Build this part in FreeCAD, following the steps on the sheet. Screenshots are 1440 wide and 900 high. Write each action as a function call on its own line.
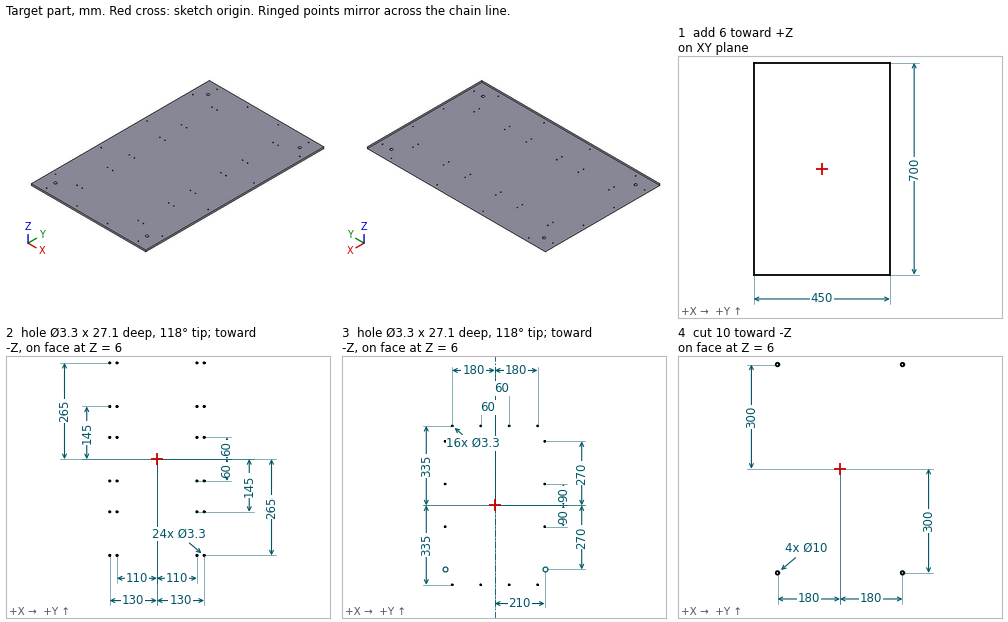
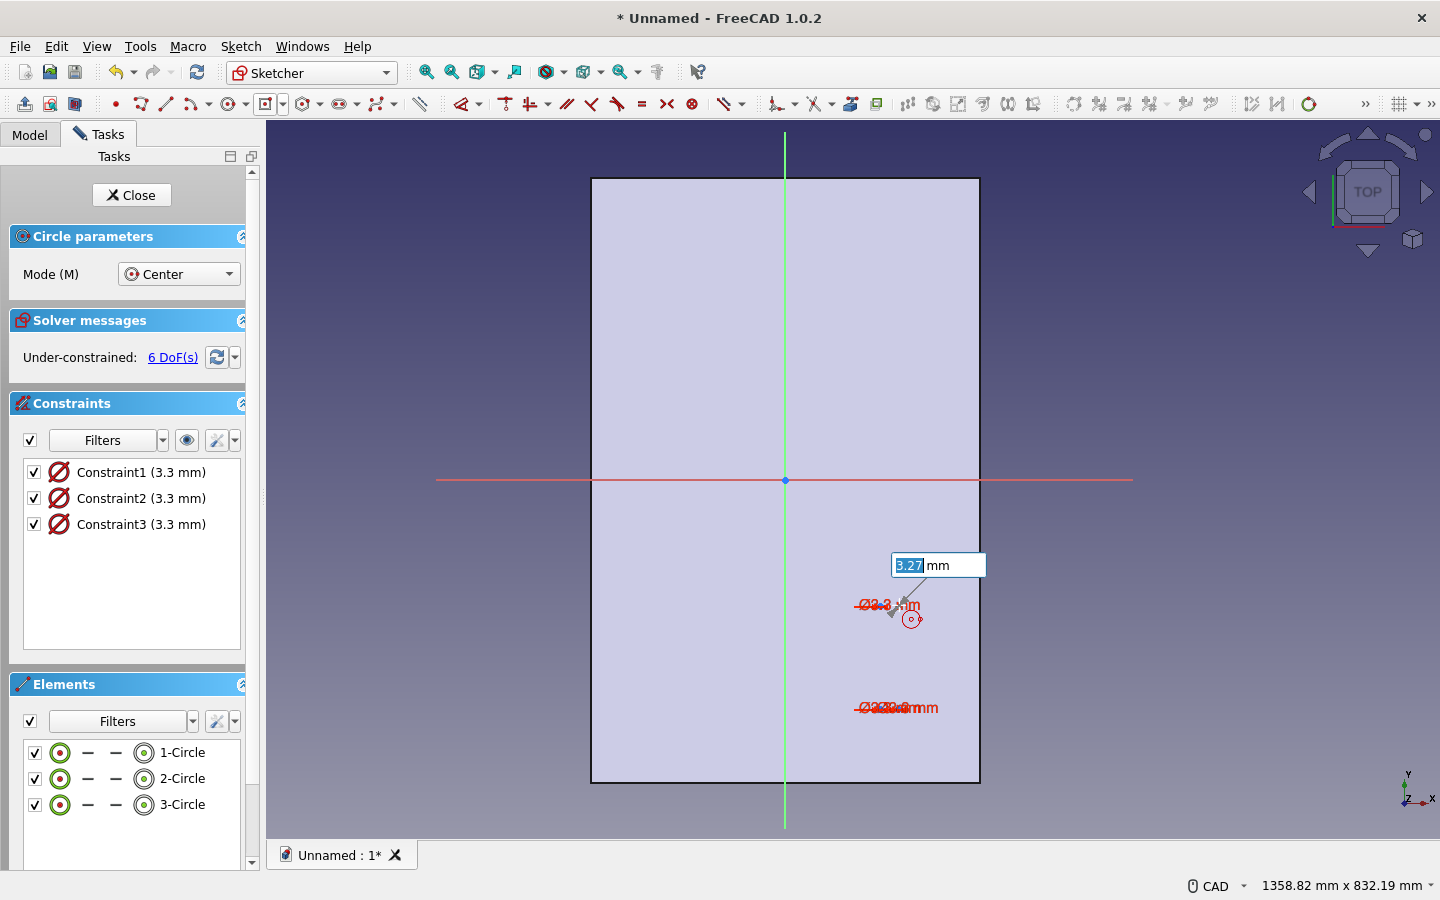
text(3.3)
key(Return)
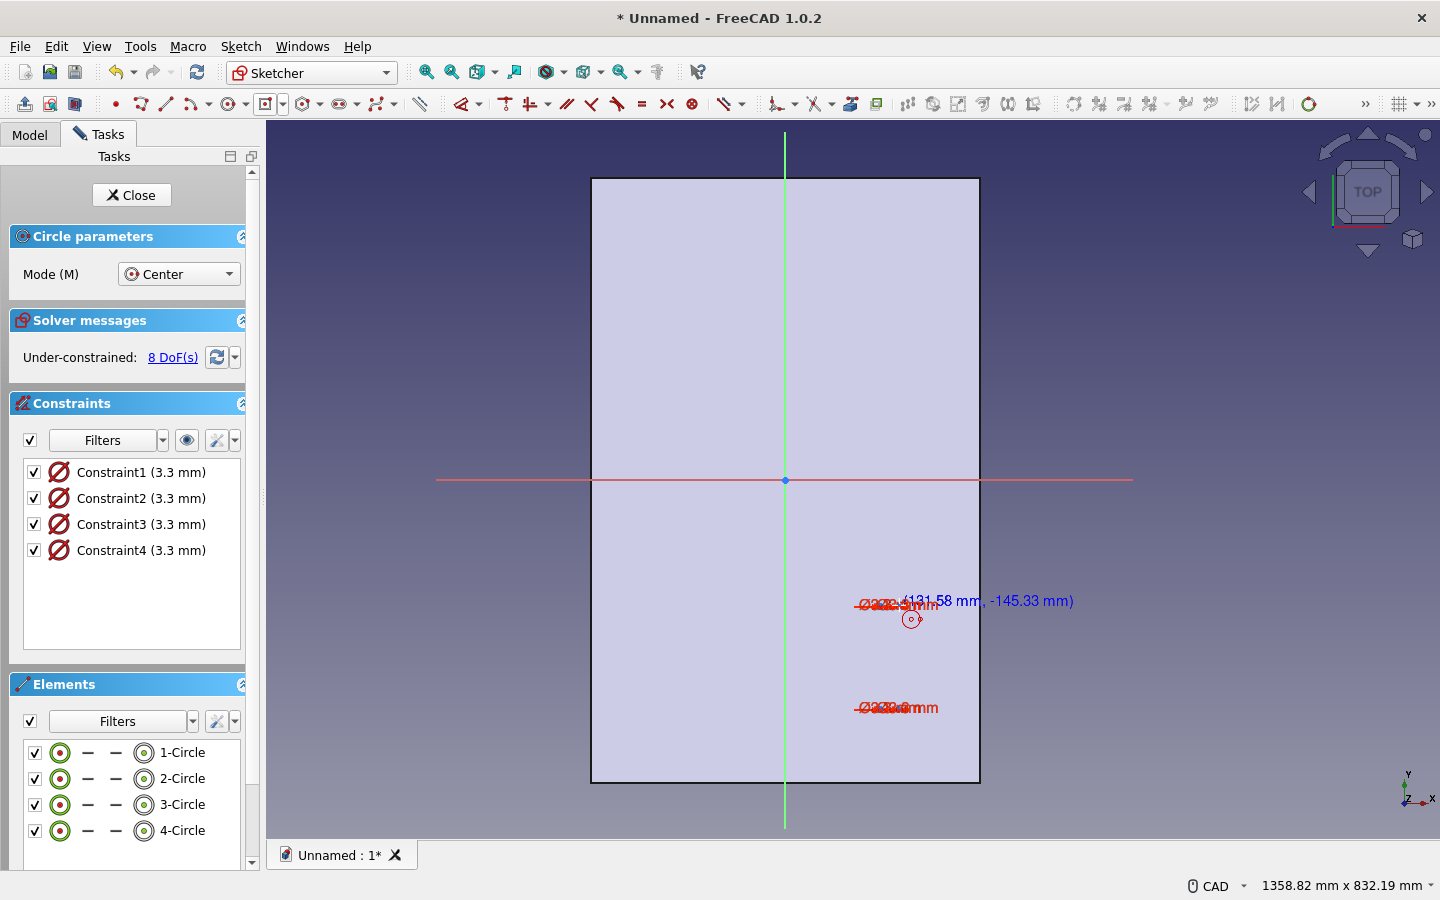
scroll(880, 532, up, 14)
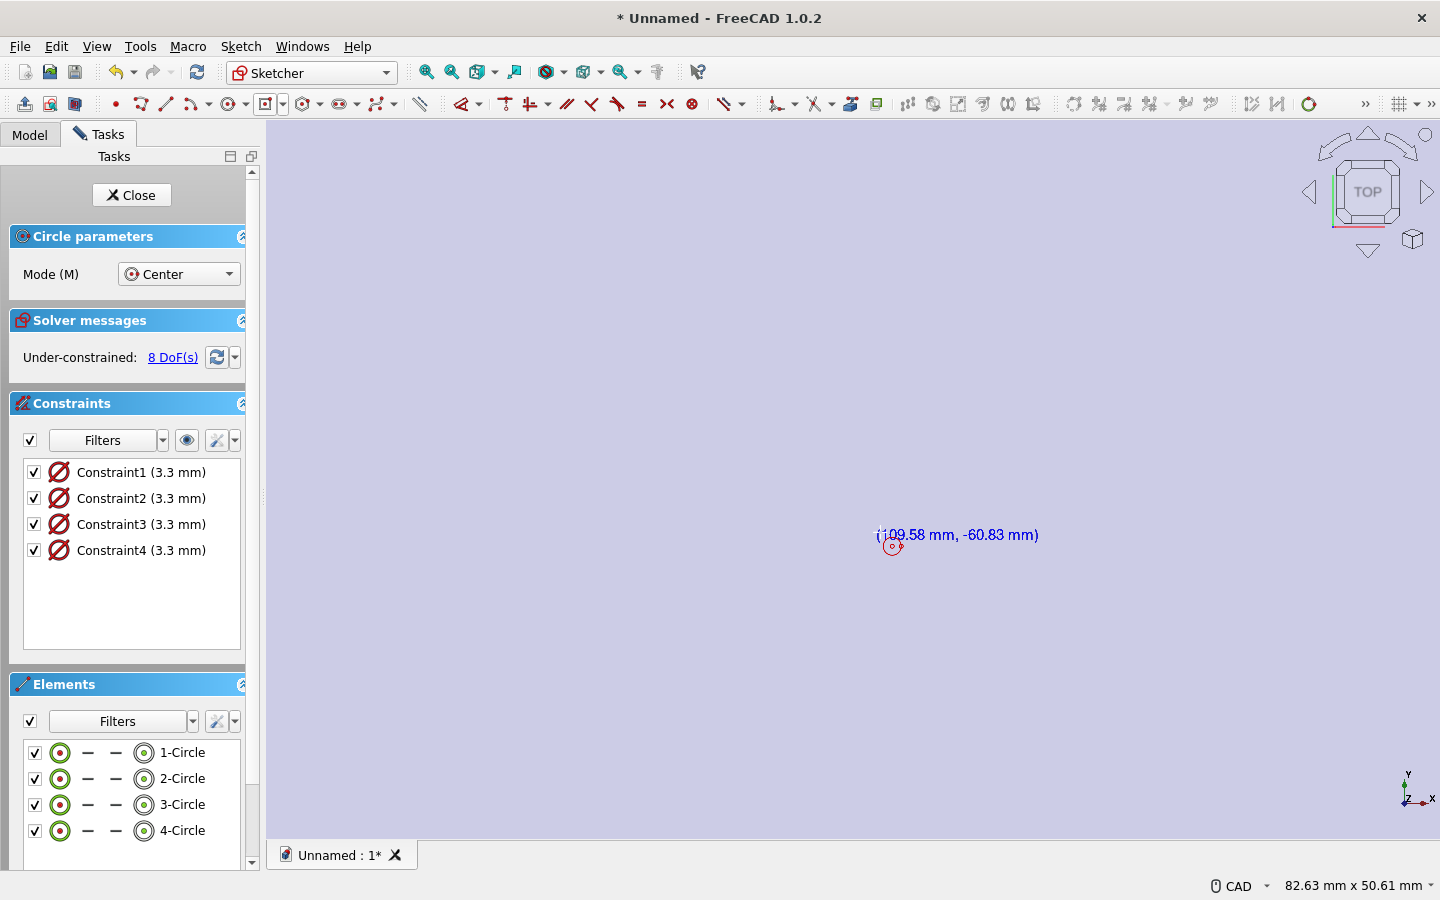
scroll(880, 532, down, 14)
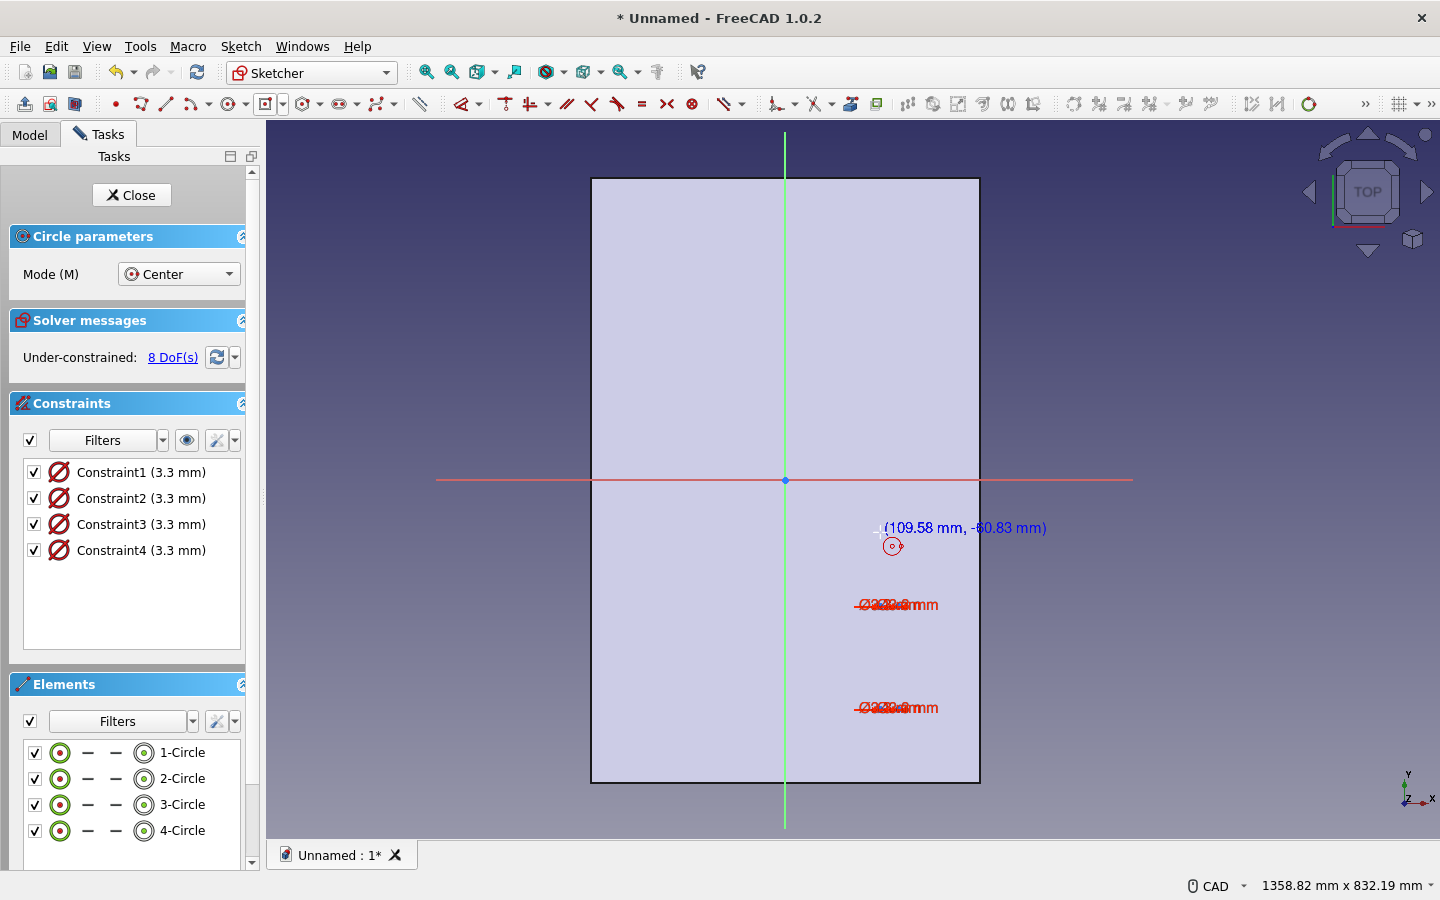
click(880, 532)
move(881, 531)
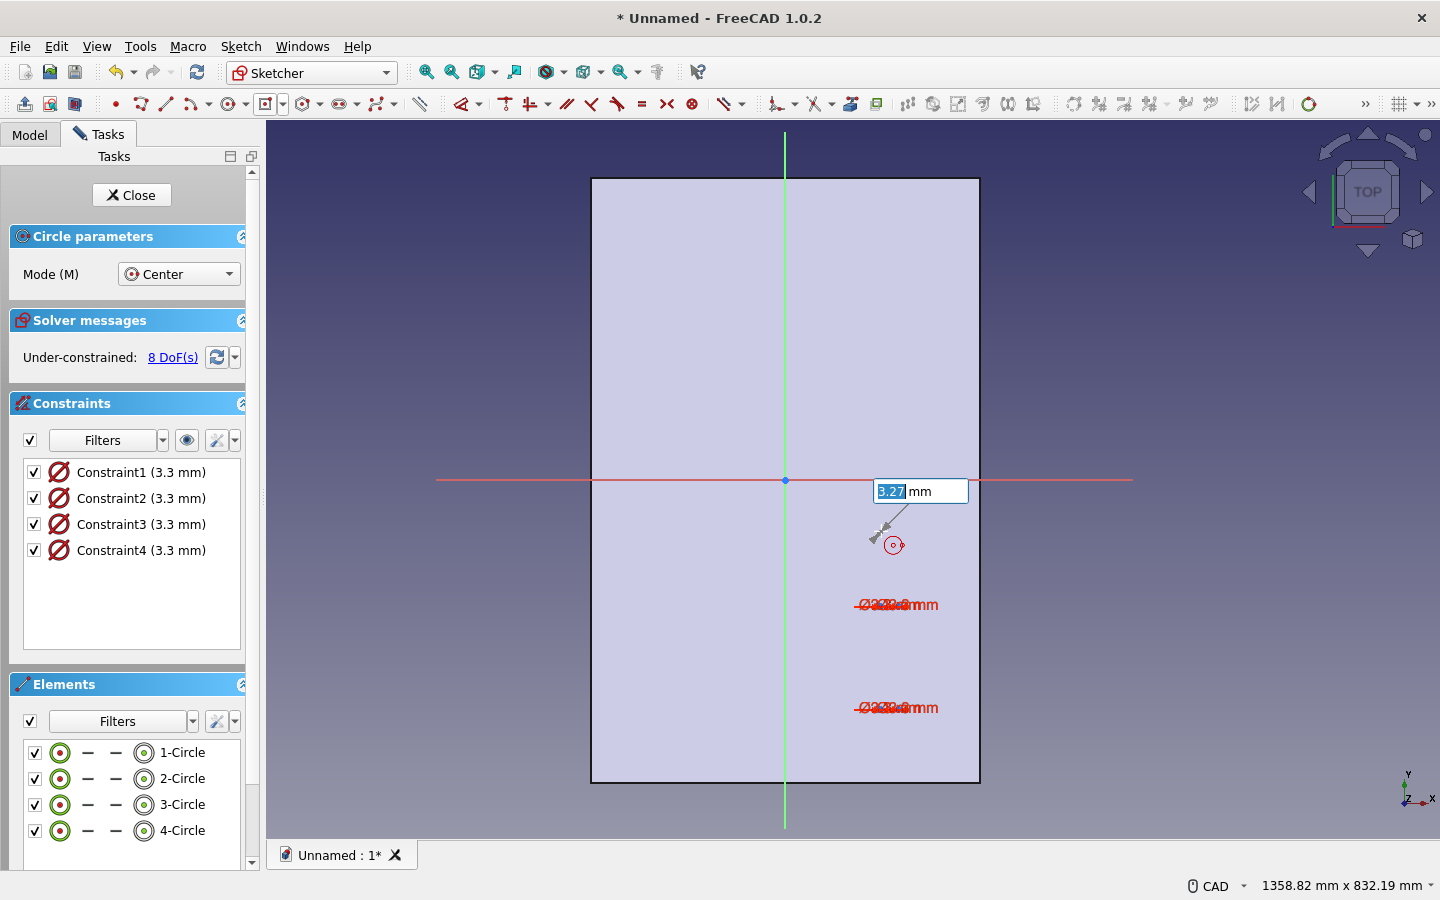
text(3.3)
key(Return)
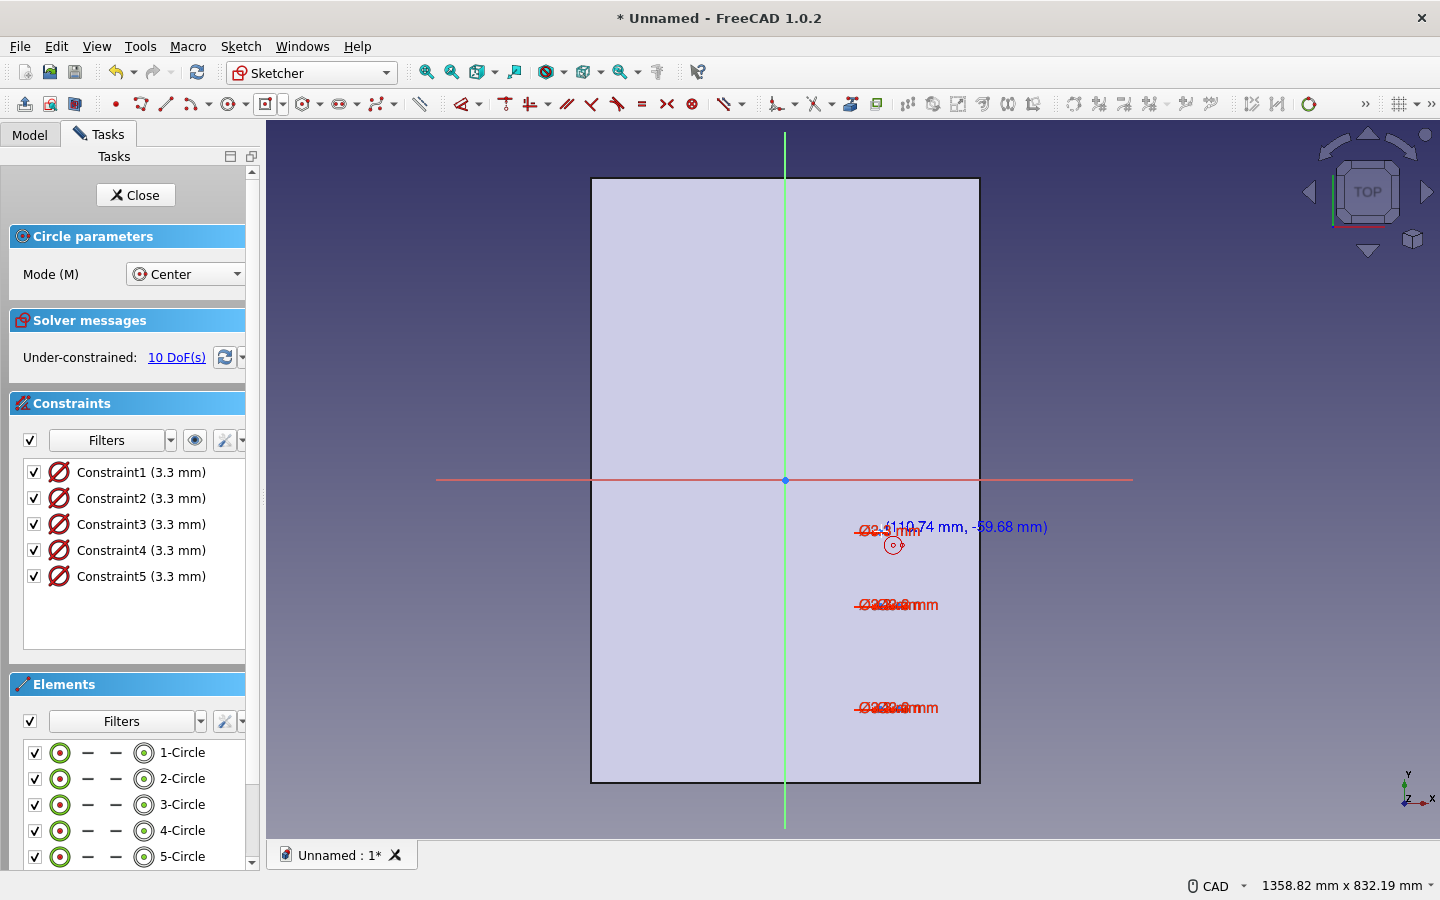
scroll(898, 532, up, 14)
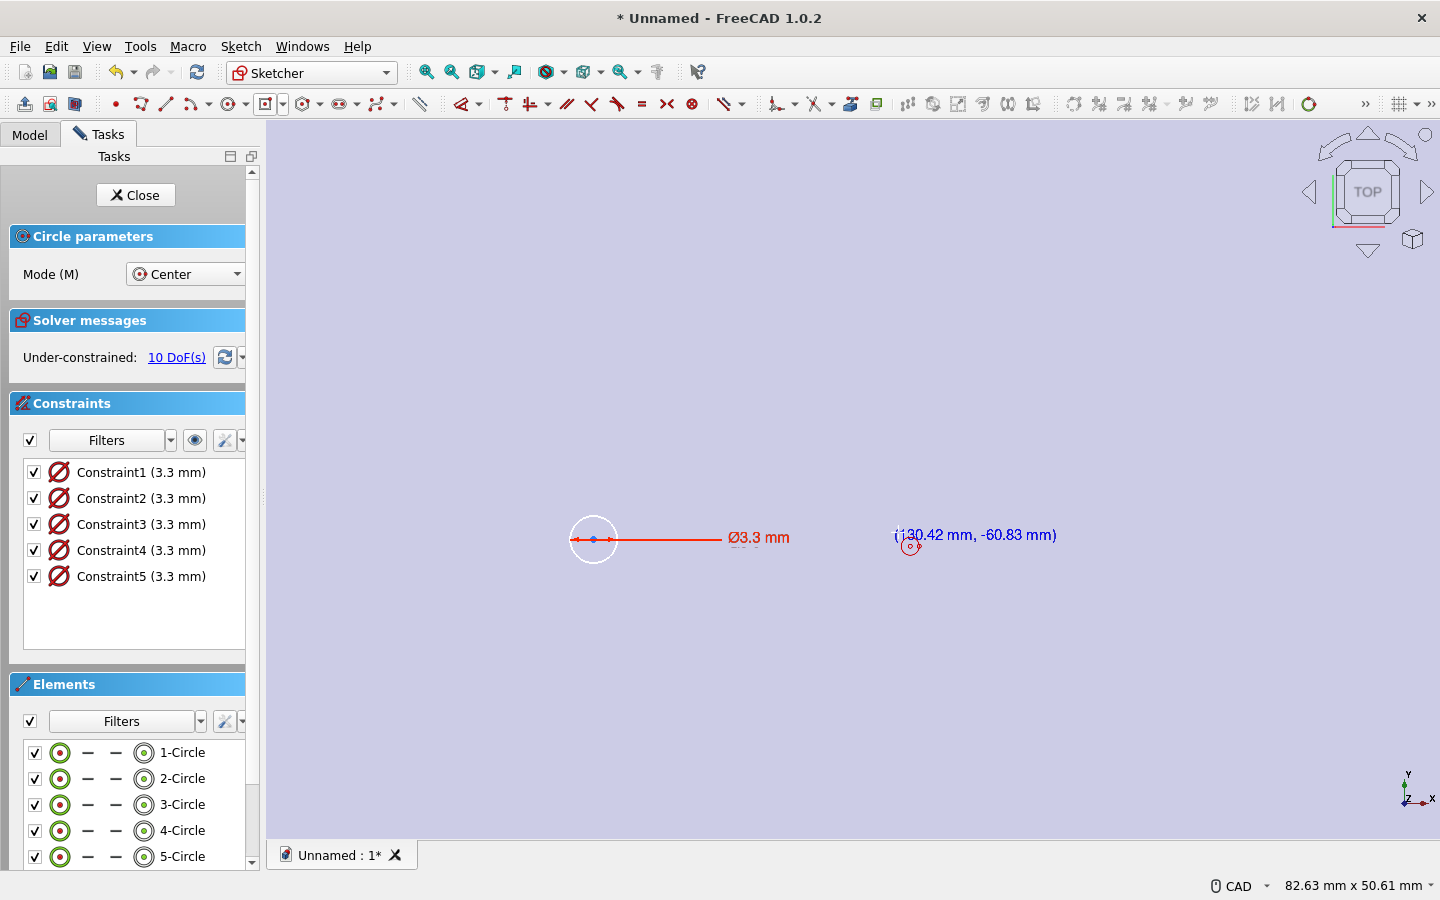
scroll(898, 532, down, 14)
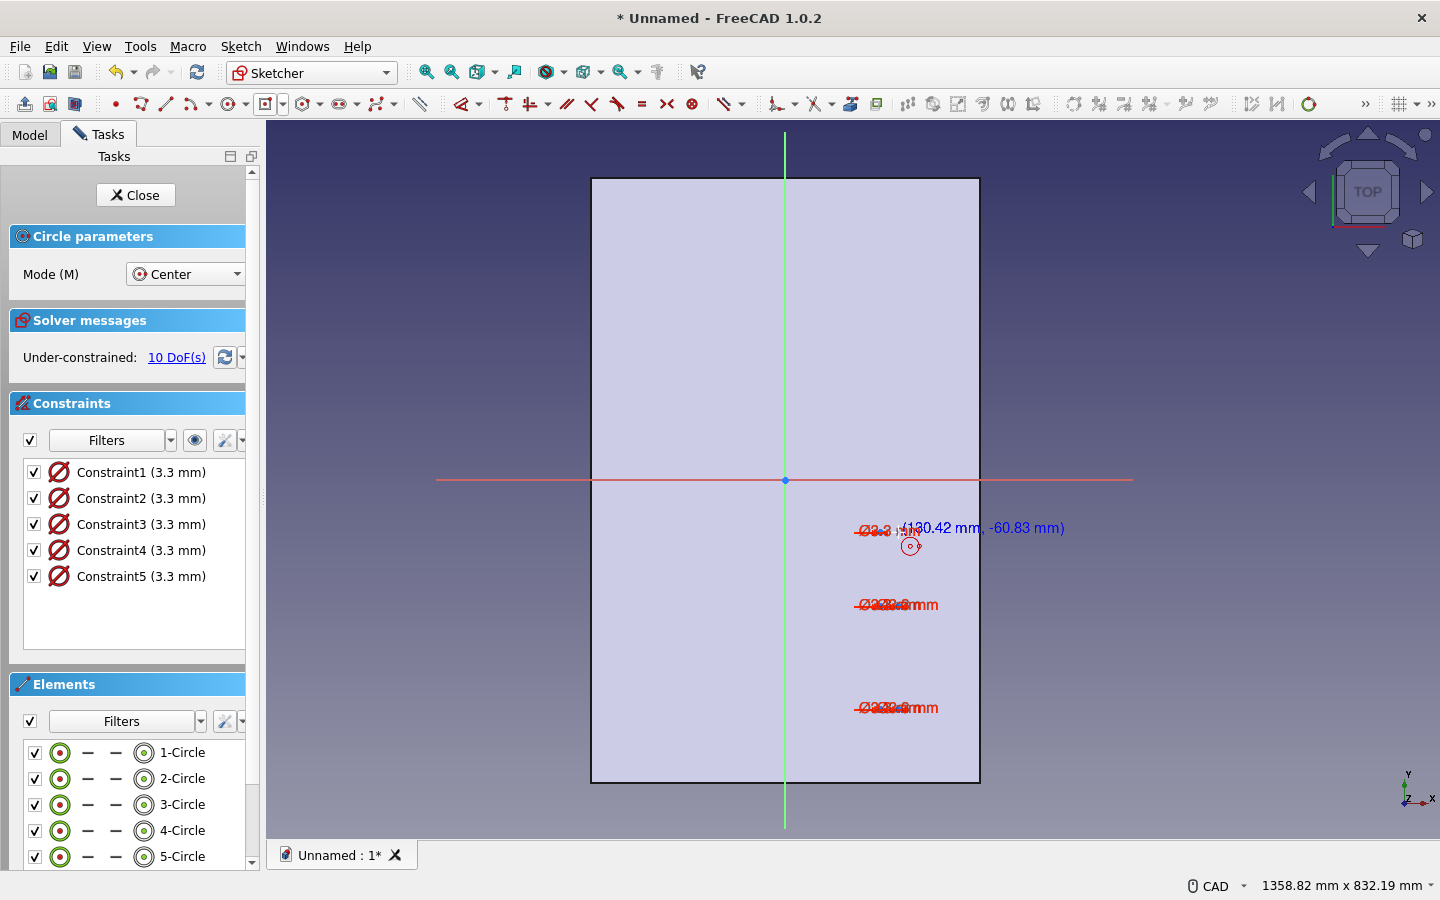
click(898, 532)
move(899, 531)